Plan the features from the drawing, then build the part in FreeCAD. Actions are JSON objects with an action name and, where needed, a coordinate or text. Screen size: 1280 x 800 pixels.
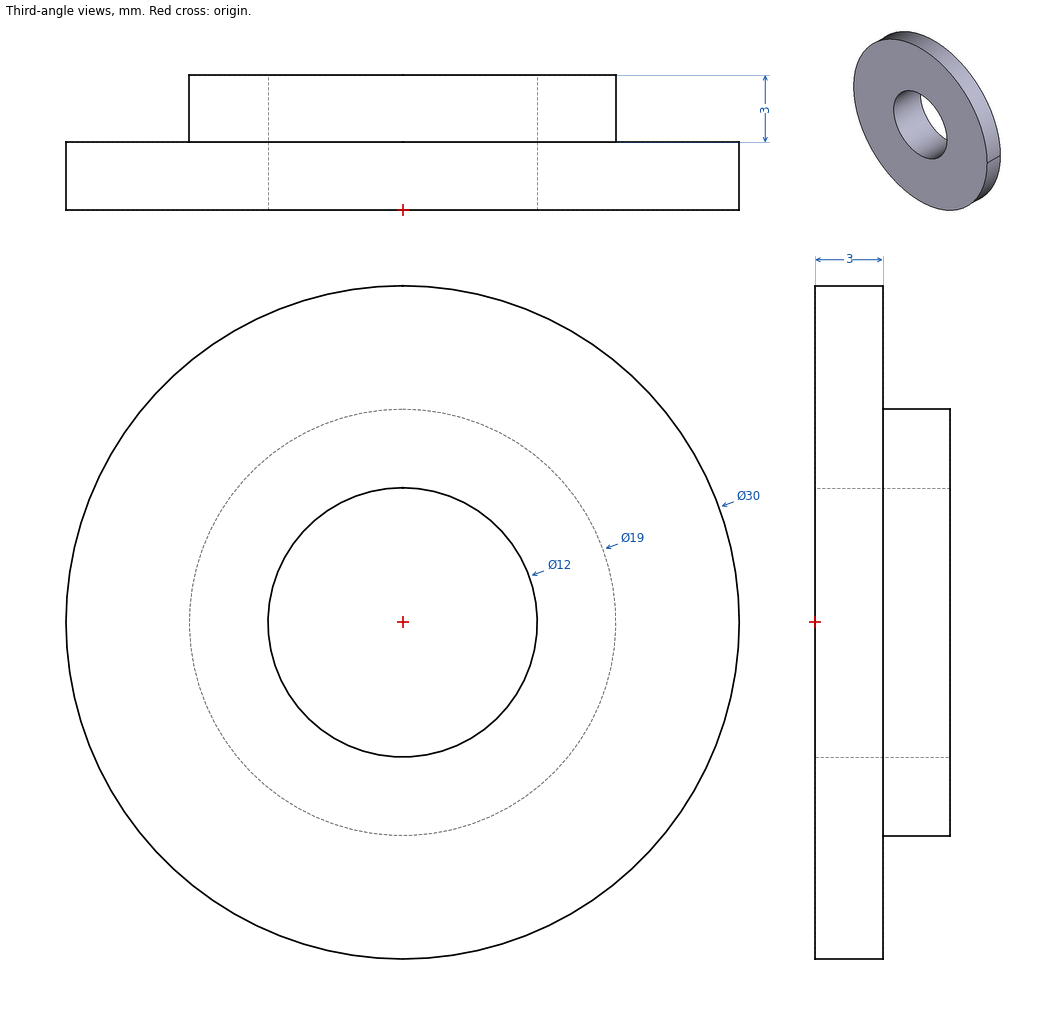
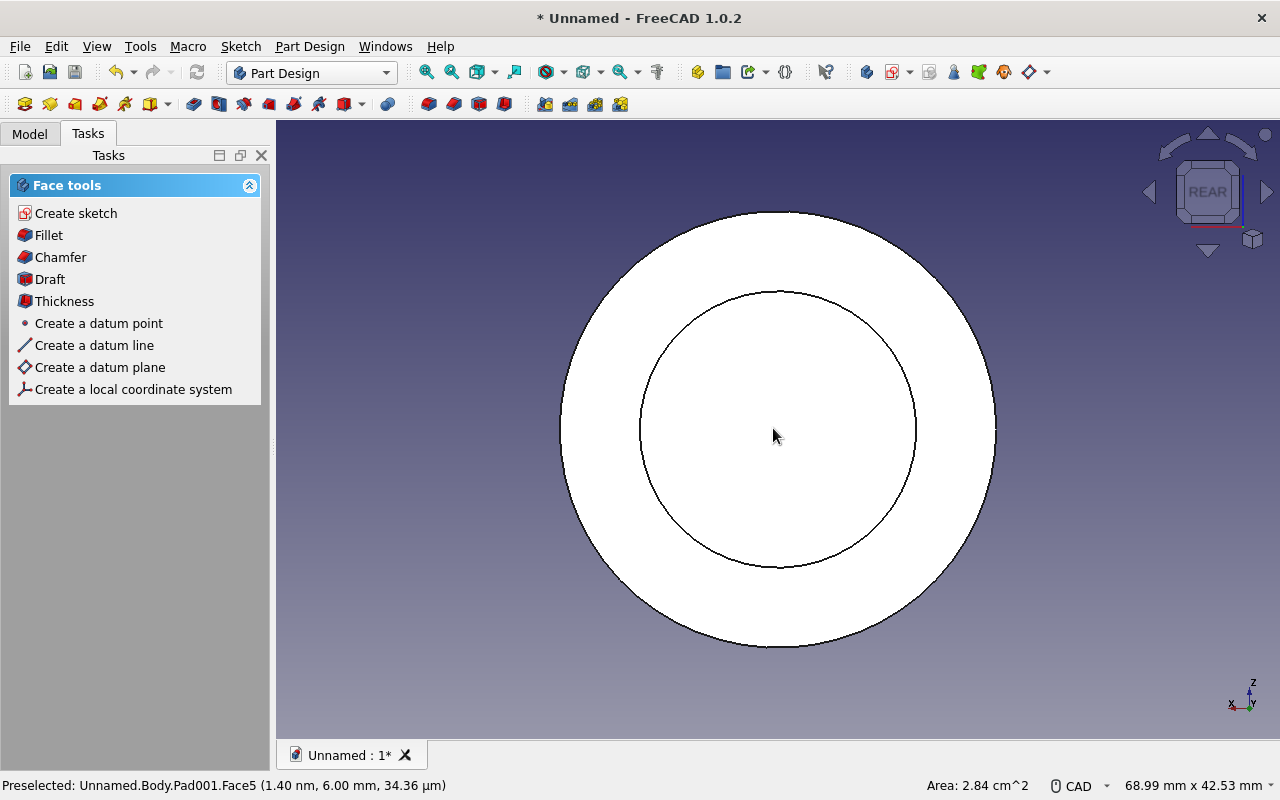
{"action": "left_click", "coordinate": [892, 72]}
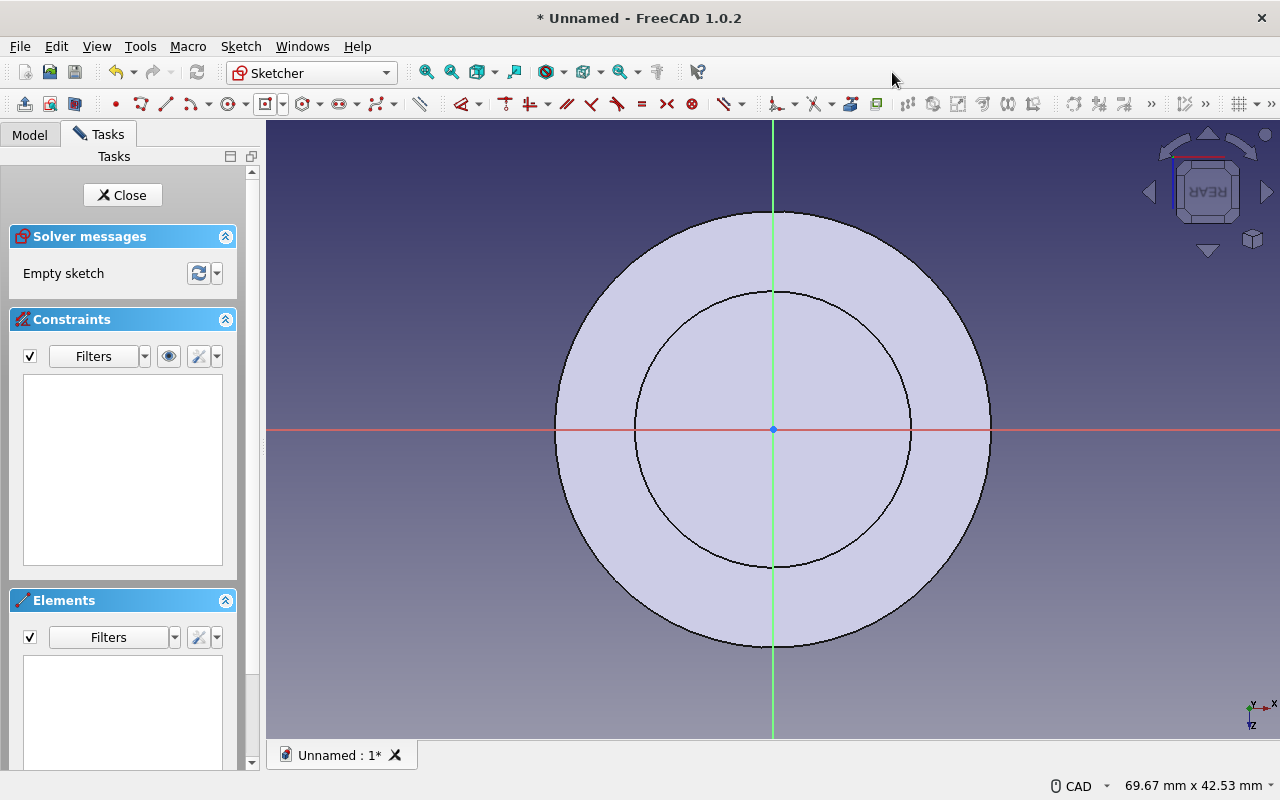
{"action": "scroll", "coordinate": [829, 429], "scroll_direction": "up", "scroll_amount": 4}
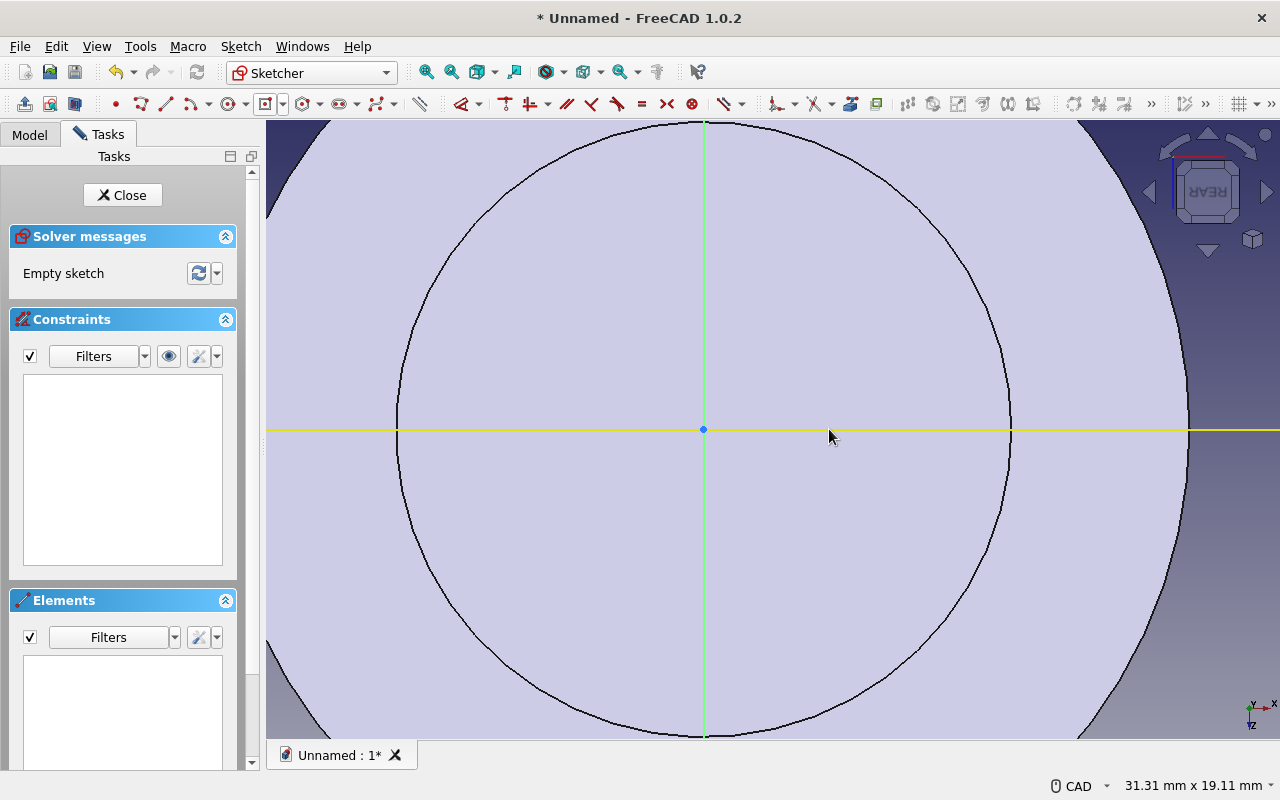
{"action": "left_click", "coordinate": [228, 104]}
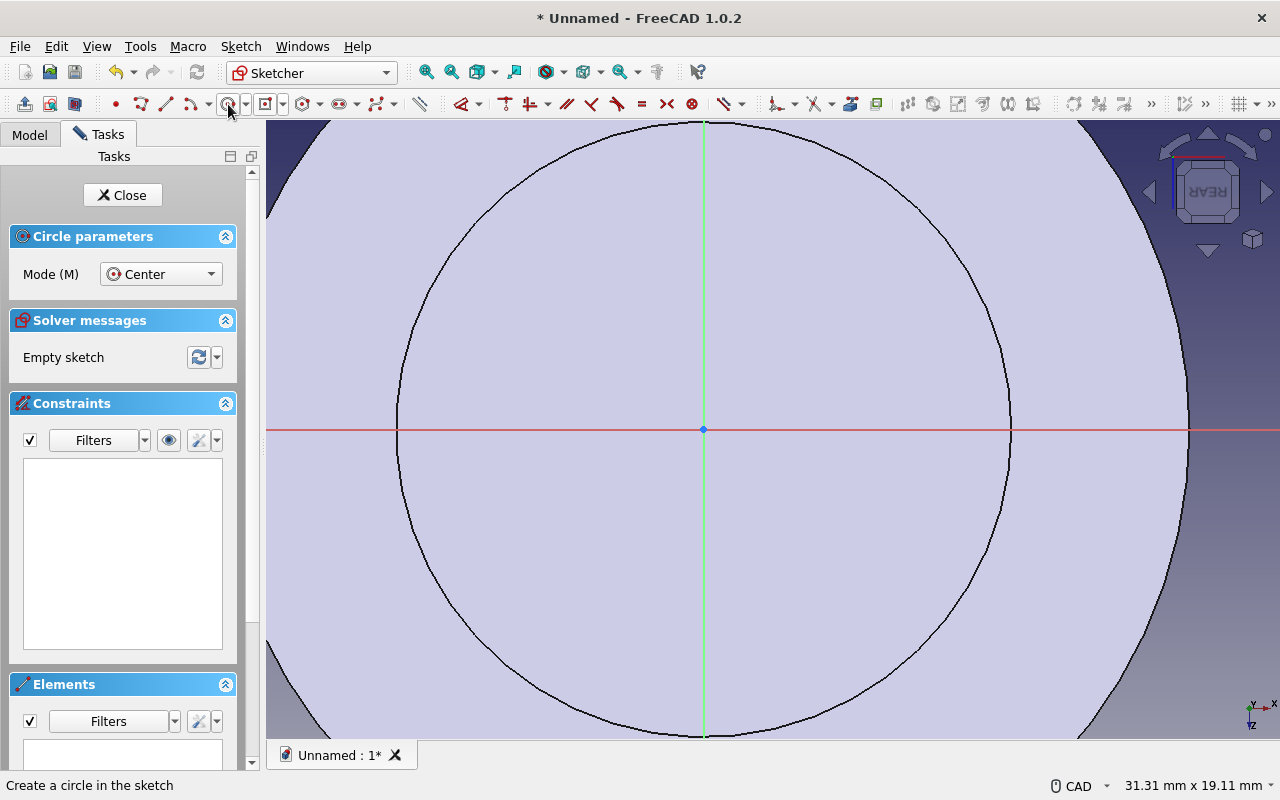
{"action": "left_click", "coordinate": [704, 429]}
{"action": "left_click", "coordinate": [841, 292]}
{"action": "key", "text": "Escape"}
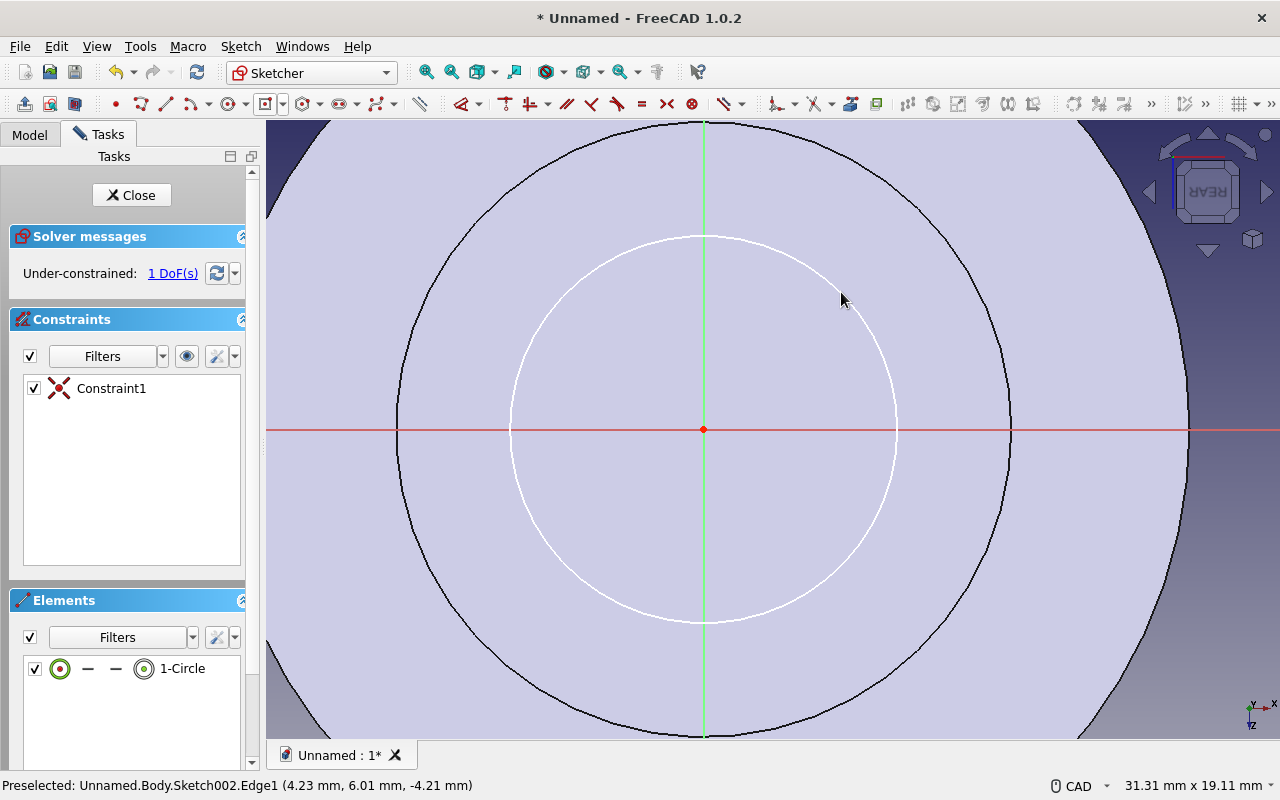
{"action": "left_click", "coordinate": [460, 104]}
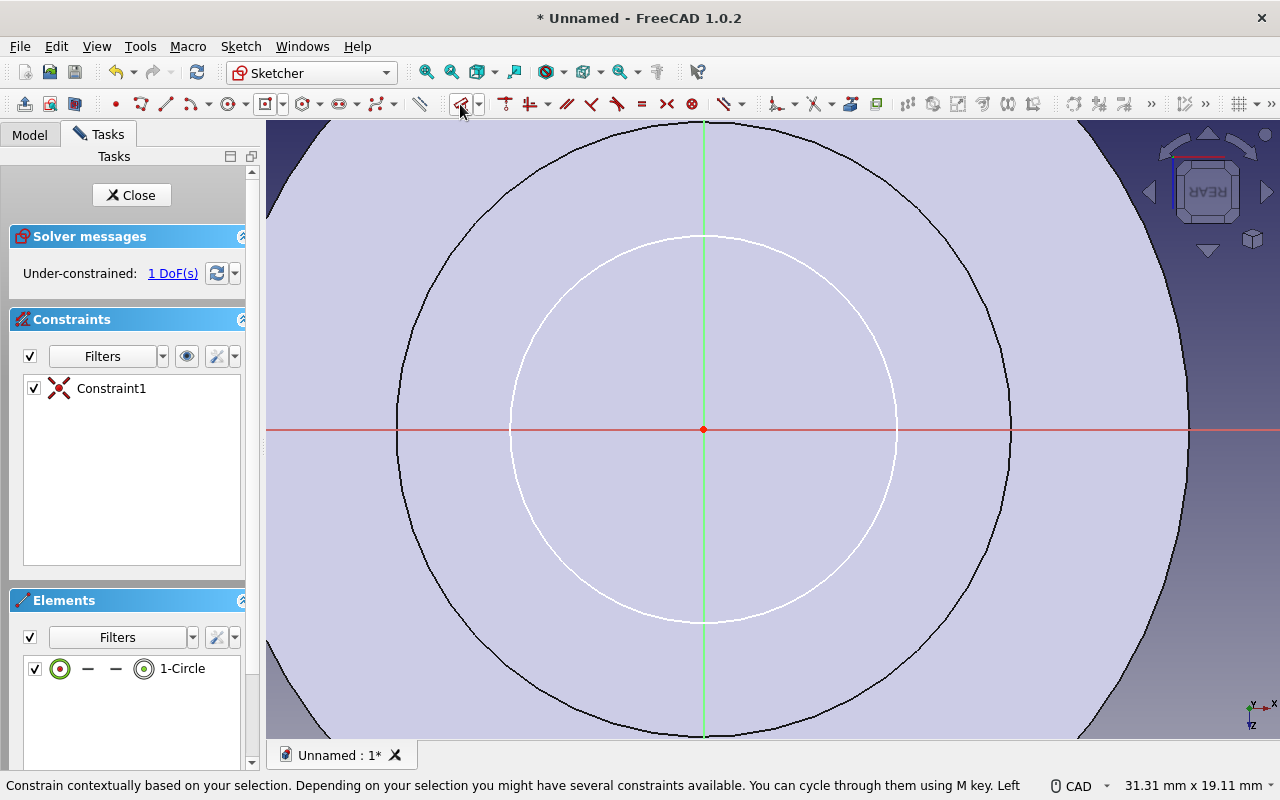
{"action": "left_click", "coordinate": [840, 292]}
{"action": "left_click", "coordinate": [863, 269]}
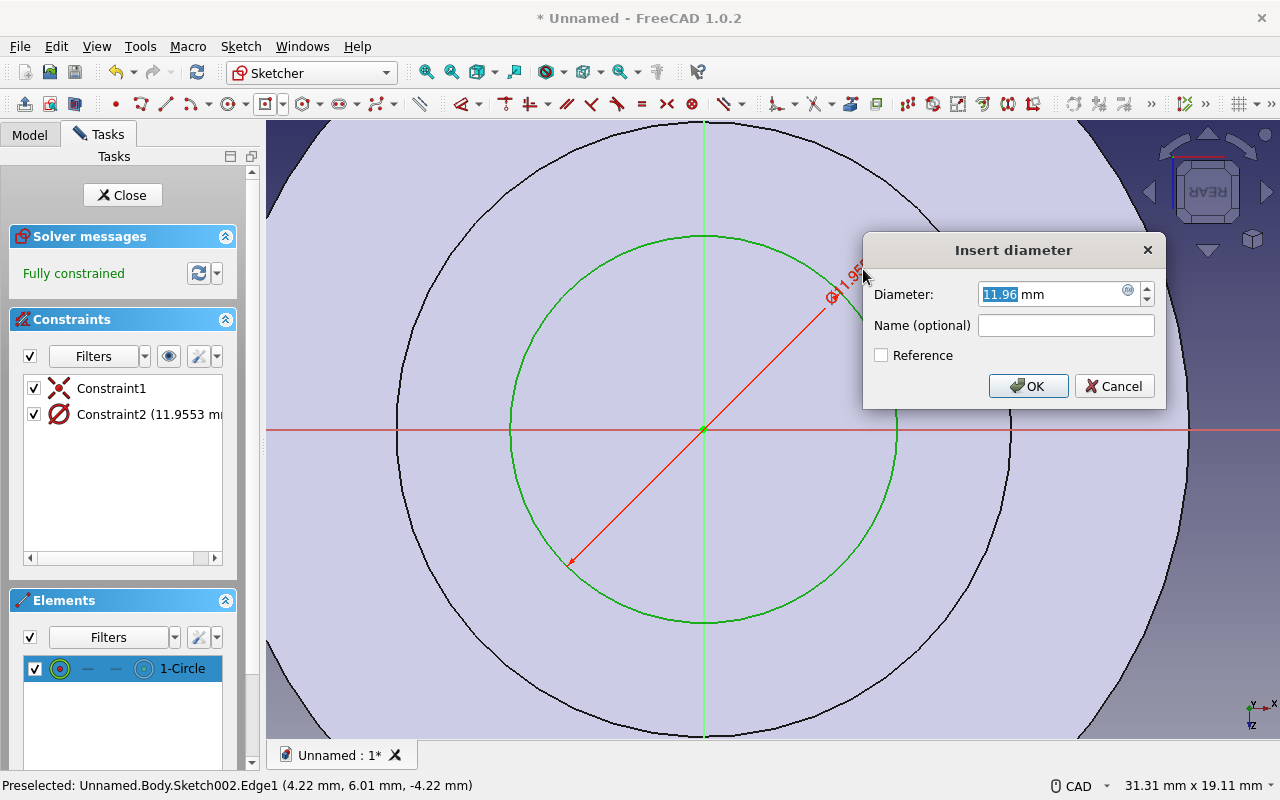
{"action": "type", "text": "12"}
{"action": "key", "text": "Return"}
{"action": "key", "text": "Escape"}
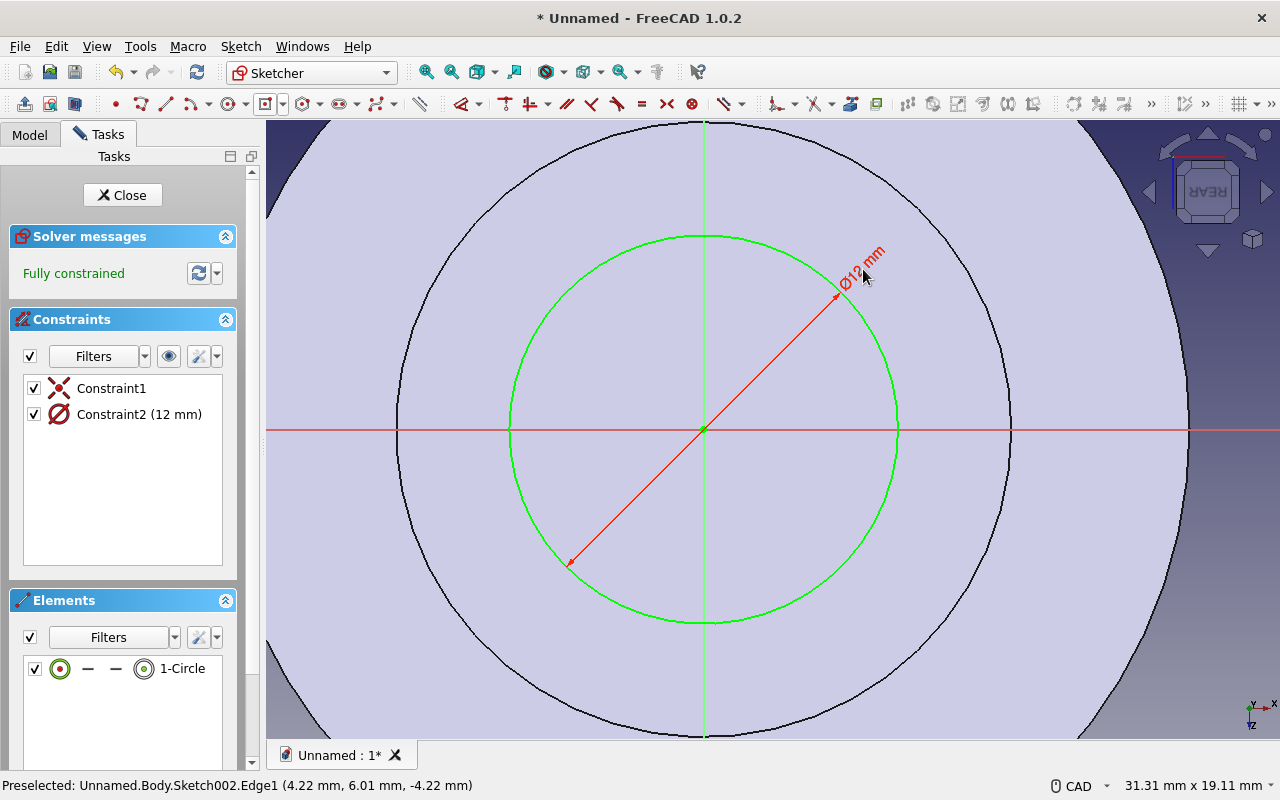
{"action": "left_click", "coordinate": [123, 195]}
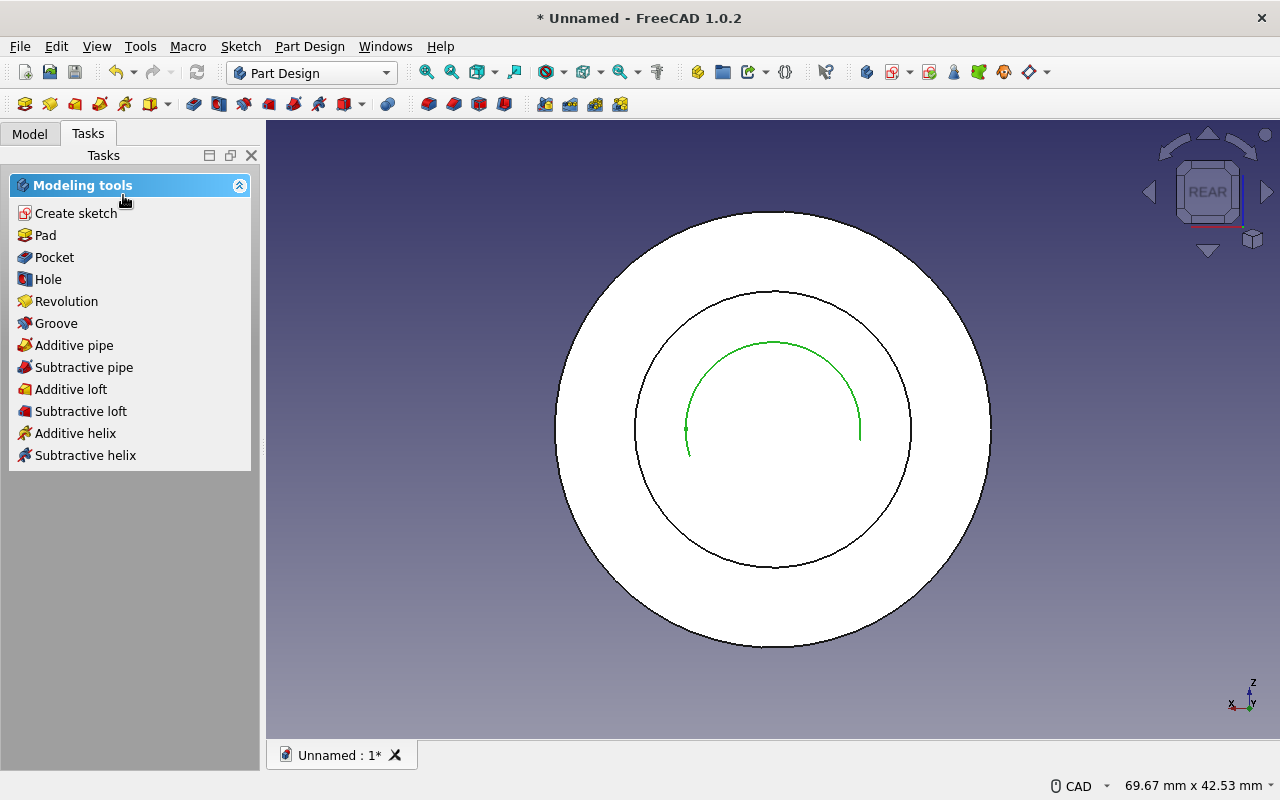
{"action": "left_click", "coordinate": [194, 104]}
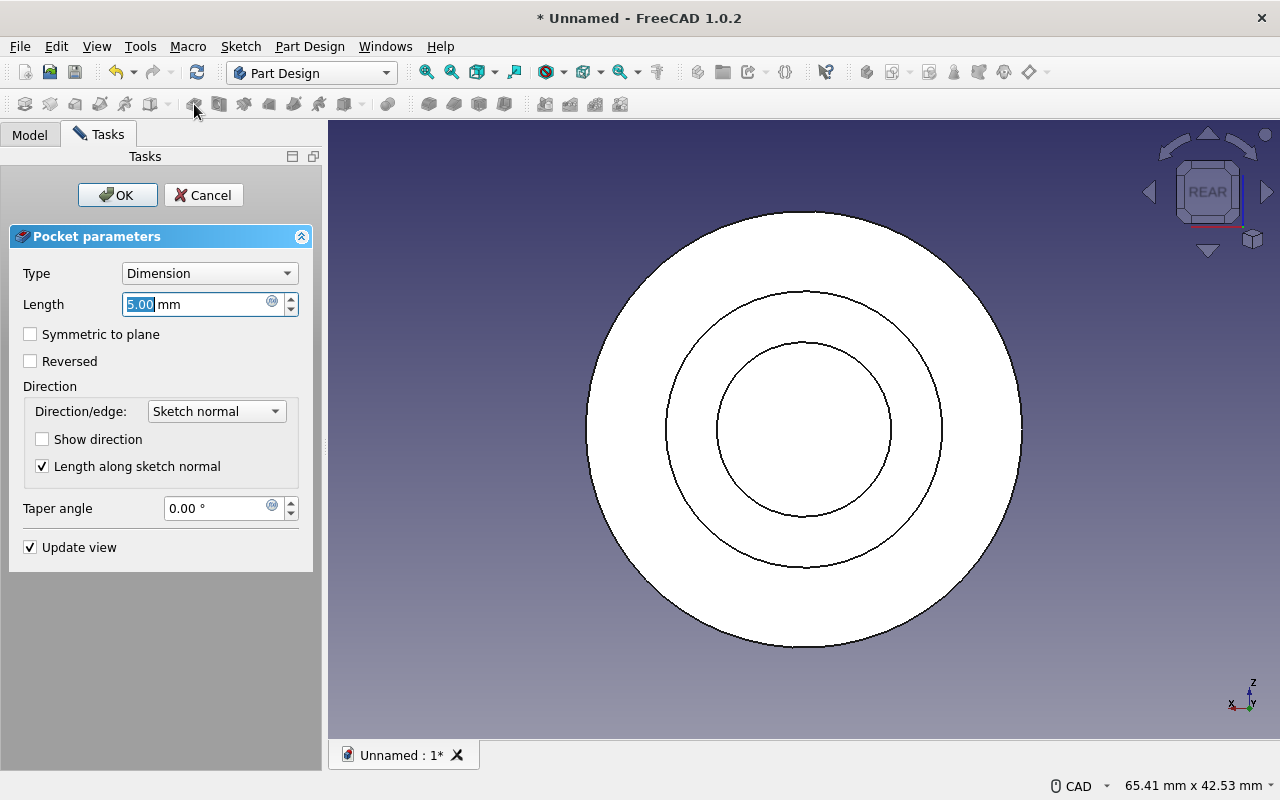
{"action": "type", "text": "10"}
{"action": "key", "text": "Tab"}